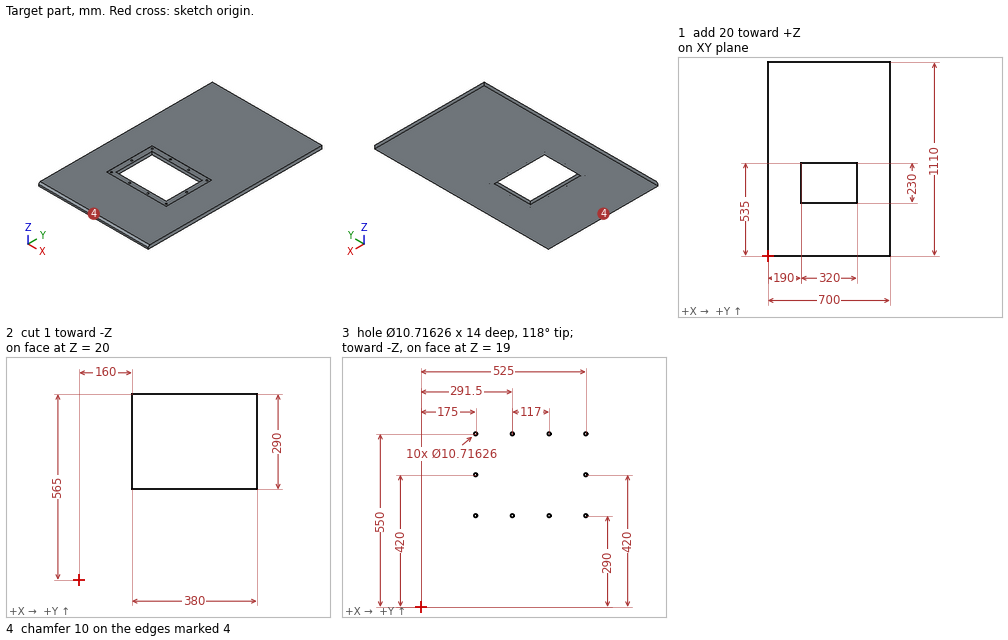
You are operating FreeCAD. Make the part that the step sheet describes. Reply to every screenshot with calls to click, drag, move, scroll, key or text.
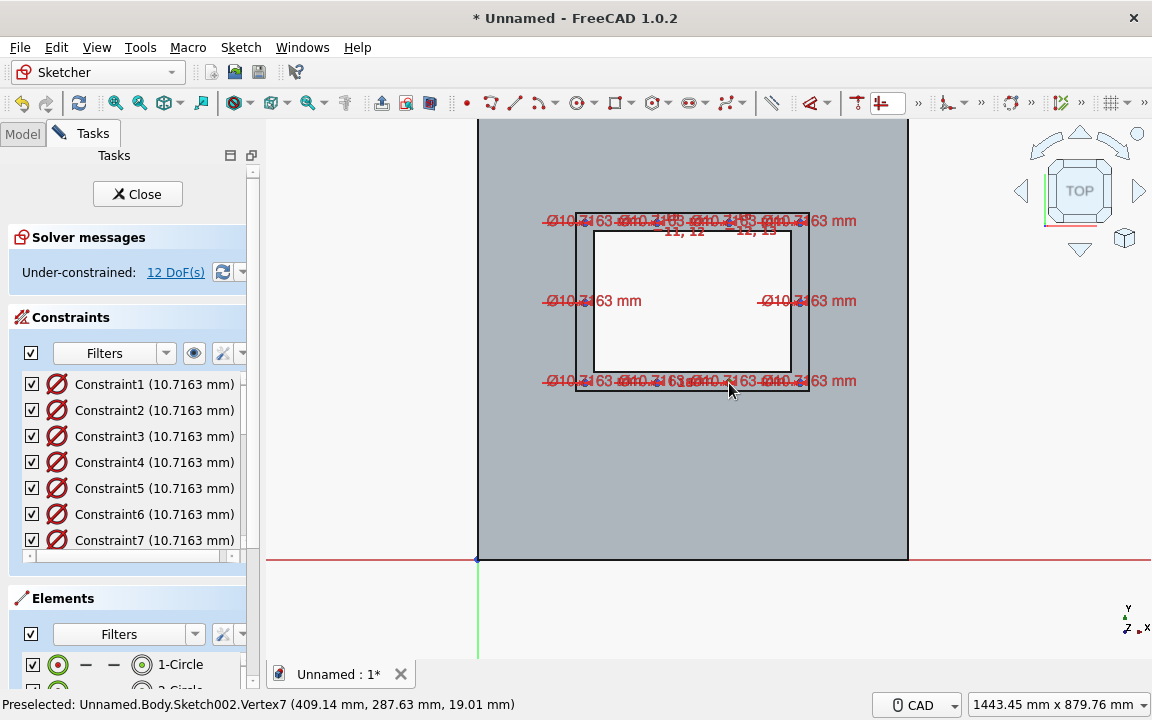
click(657, 383)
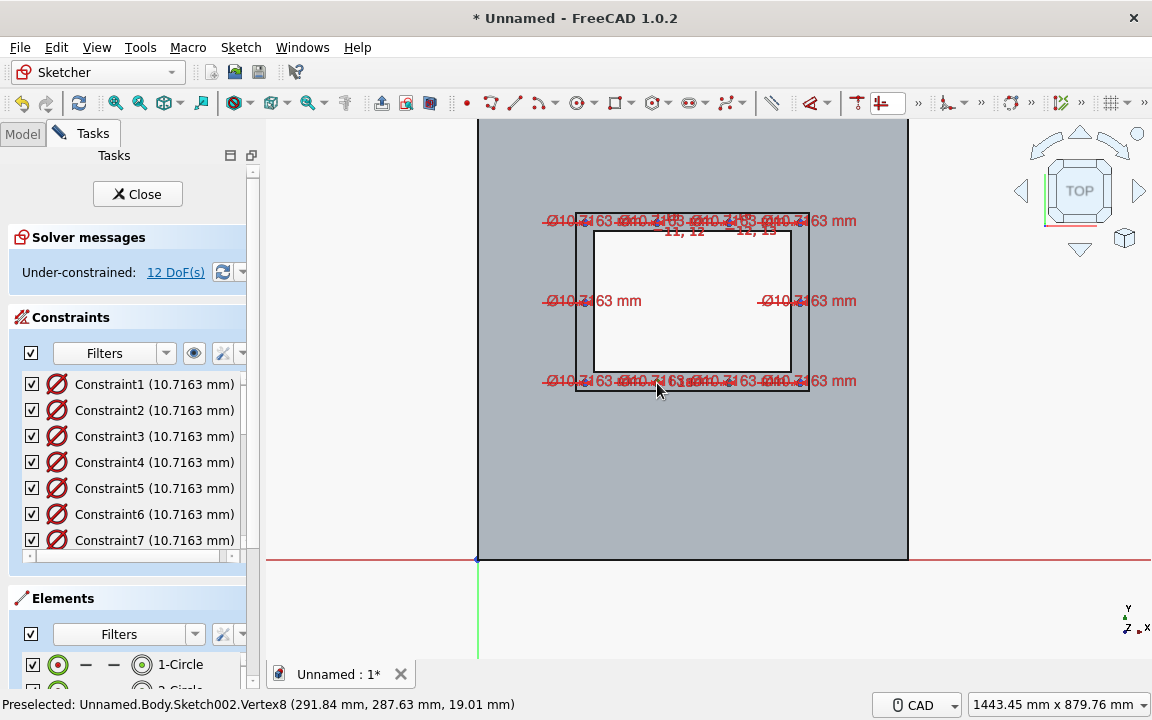
key(h)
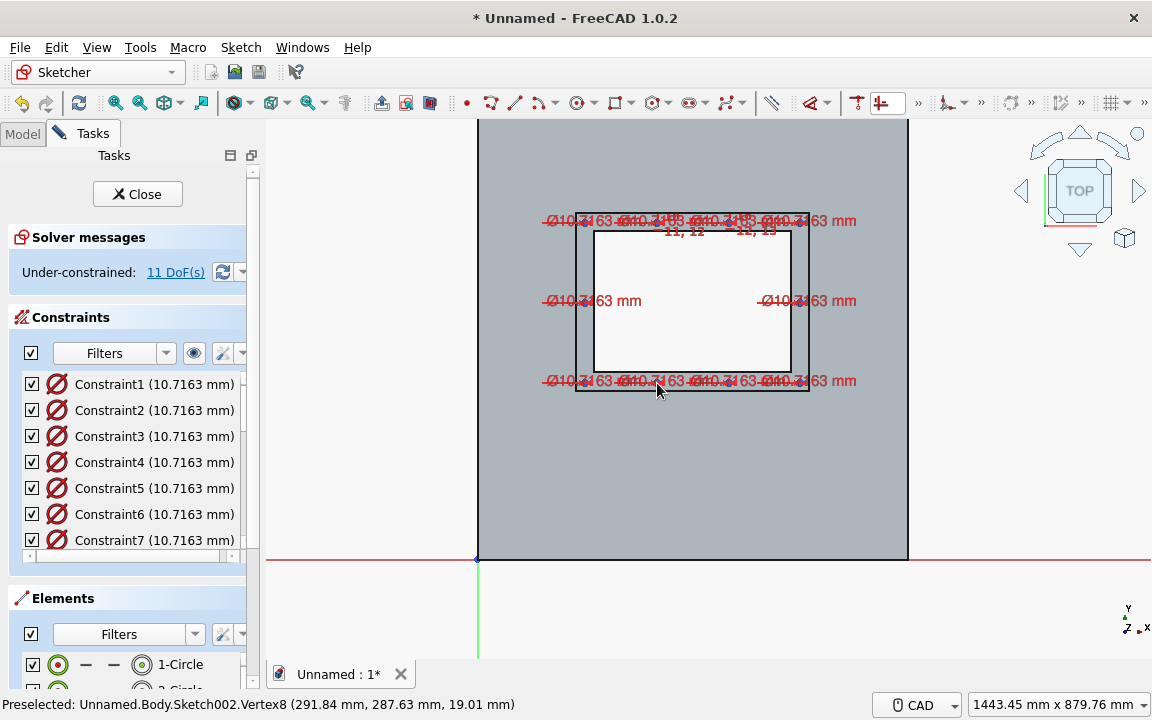
click(585, 223)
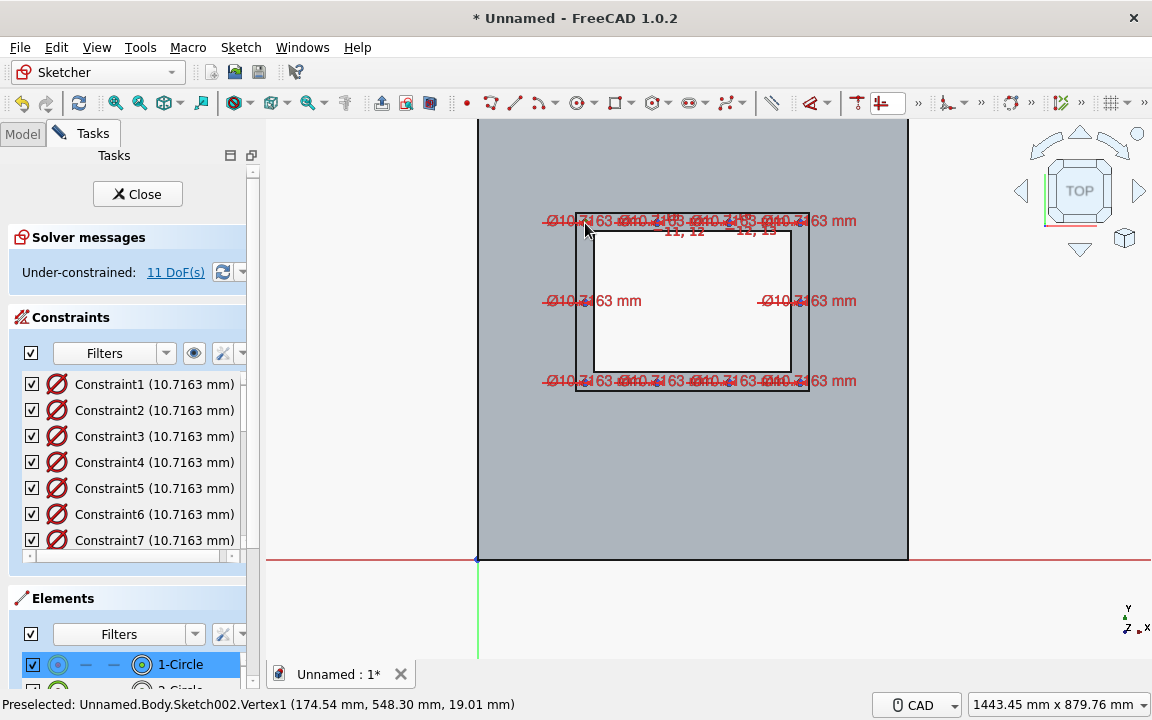
click(585, 383)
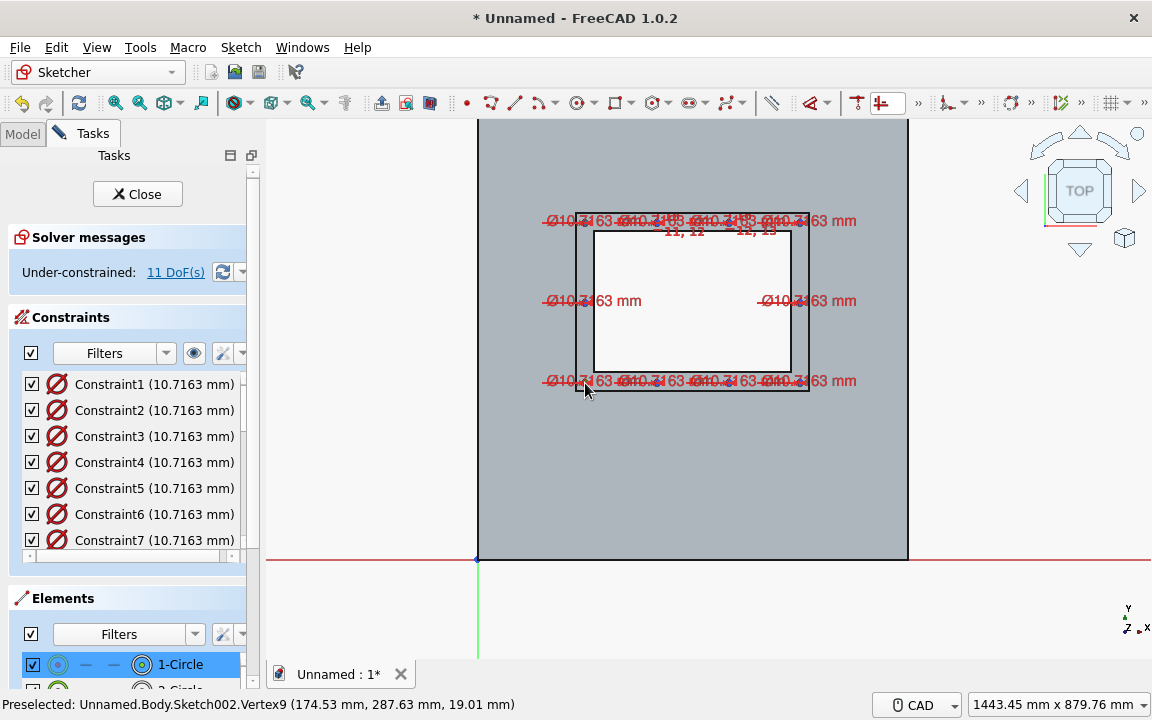
key(v)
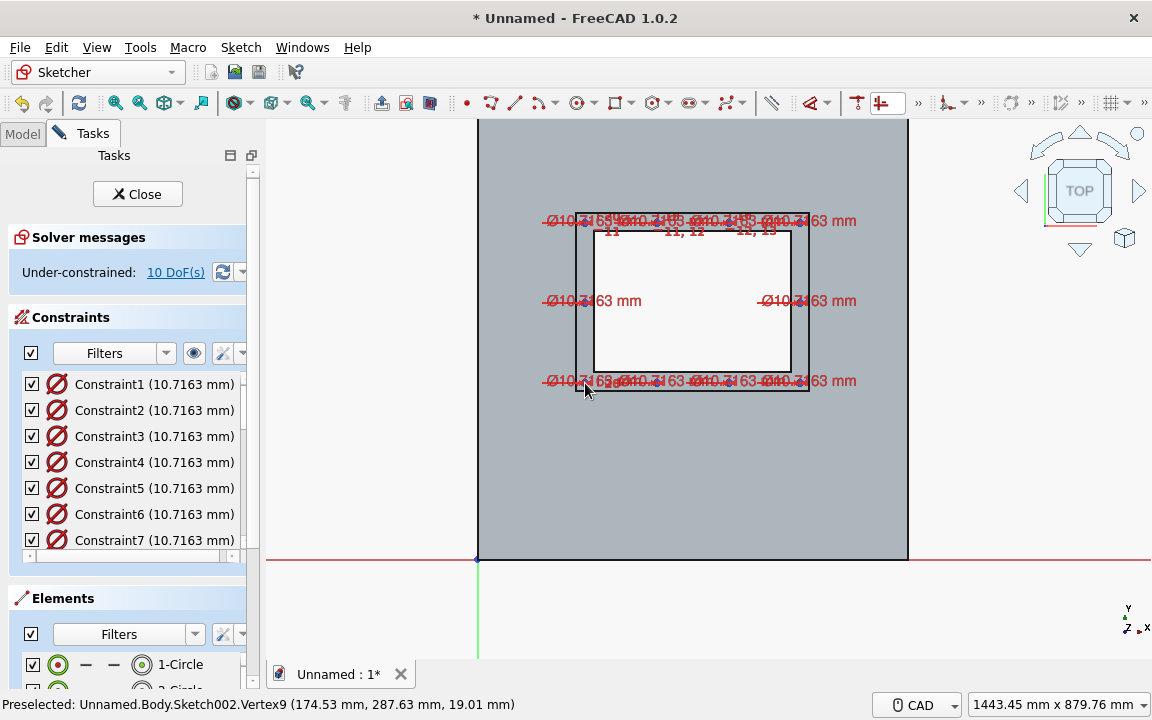
click(657, 383)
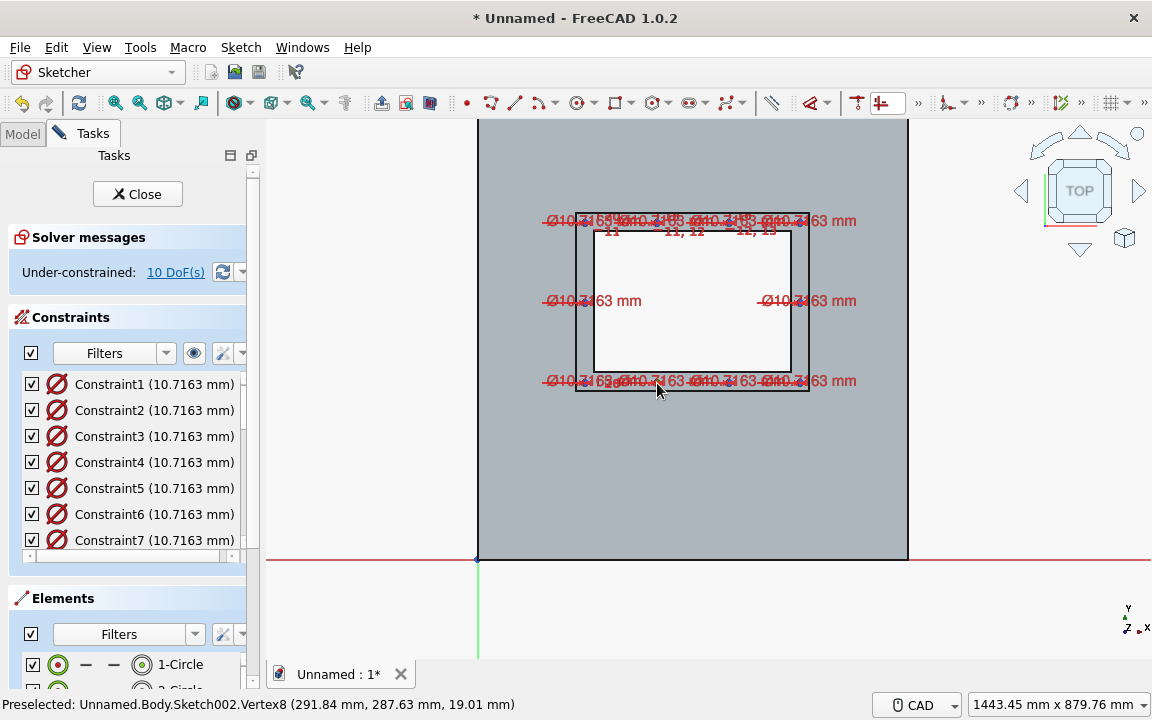
click(585, 383)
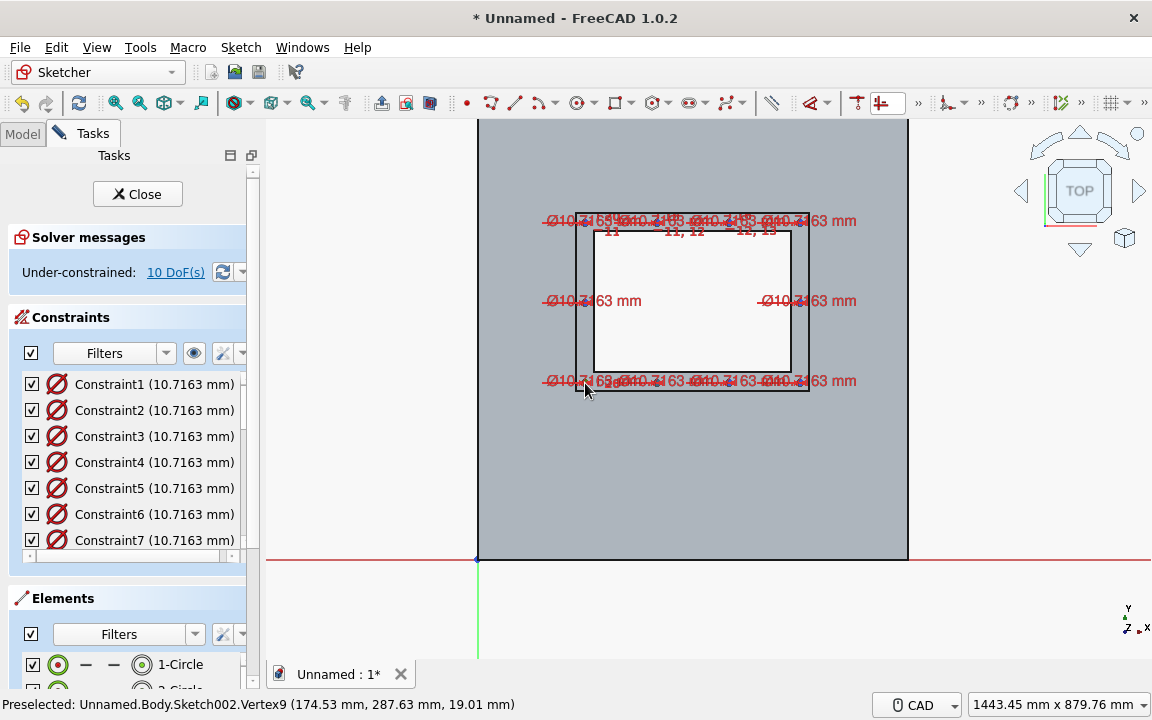
key(h)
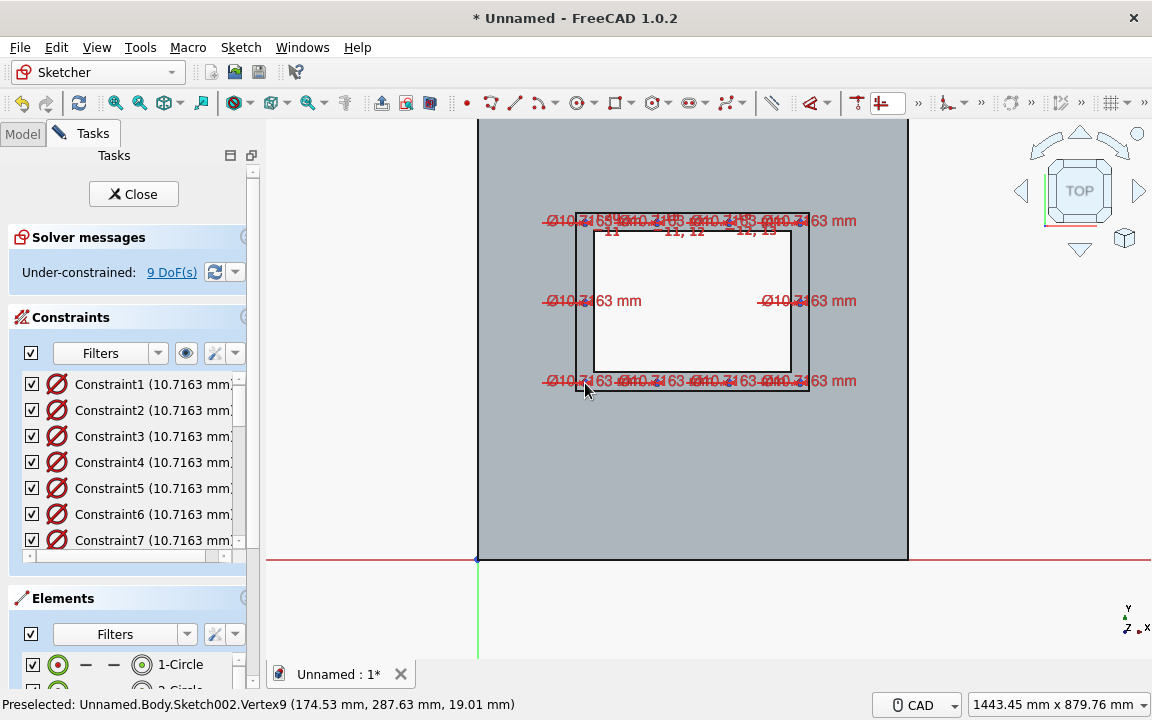
click(585, 223)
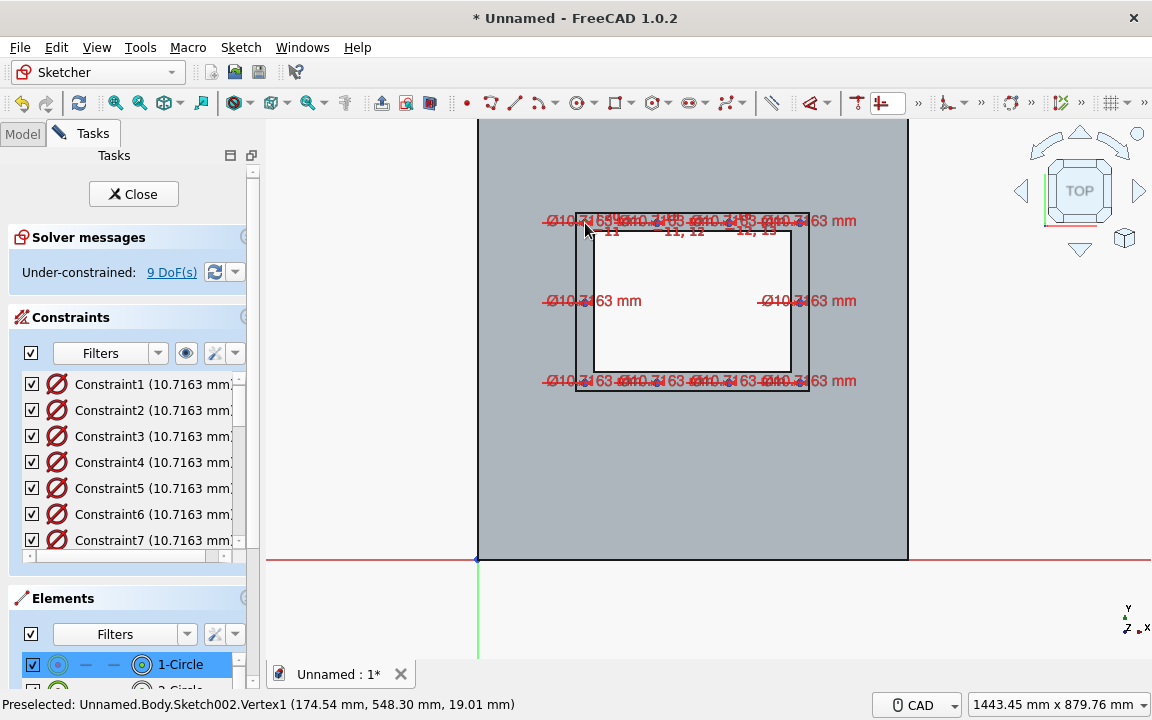
click(585, 303)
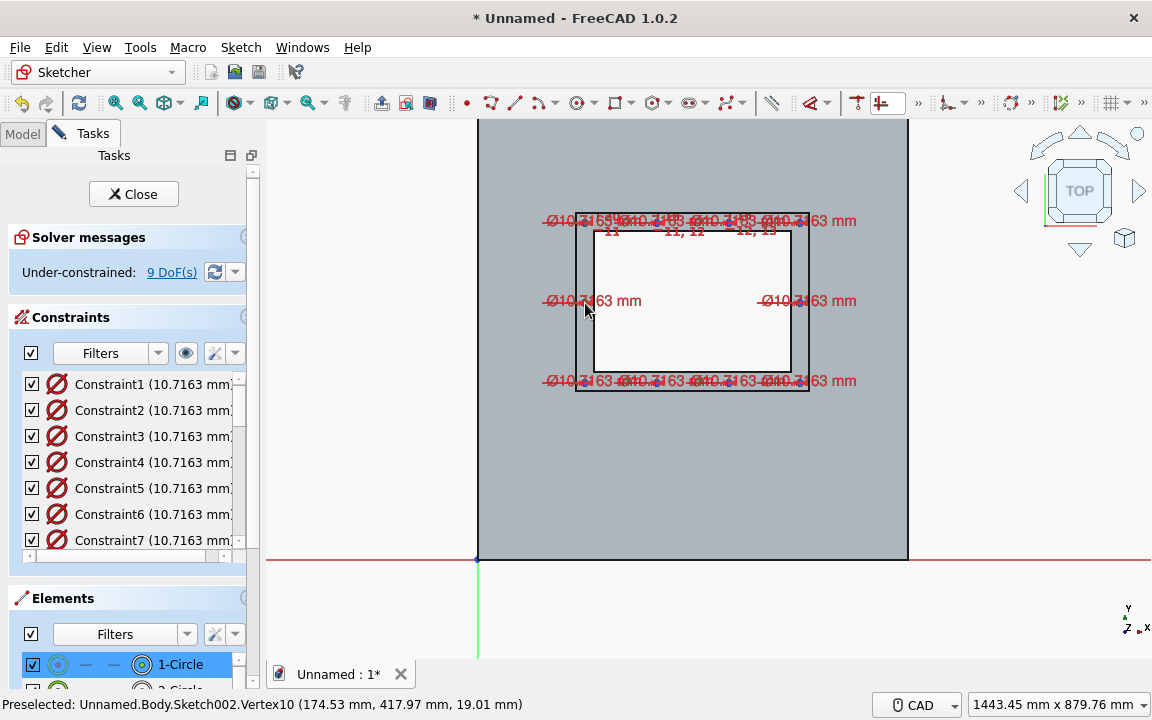
click(900, 104)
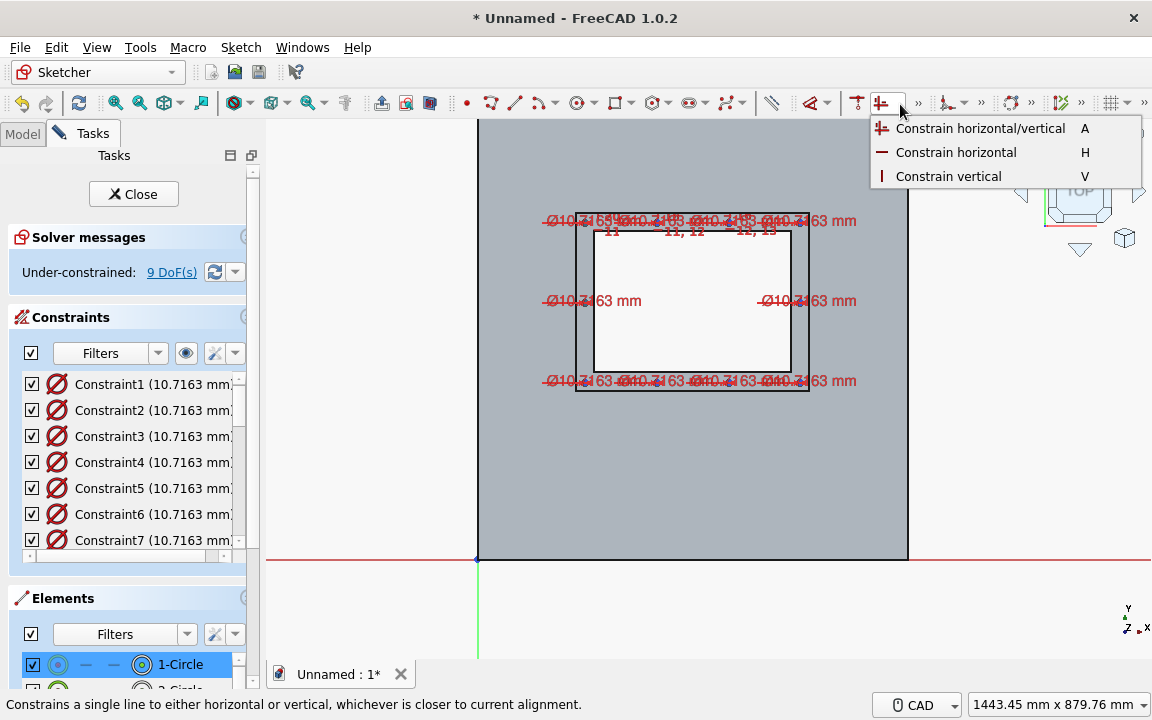
click(1006, 176)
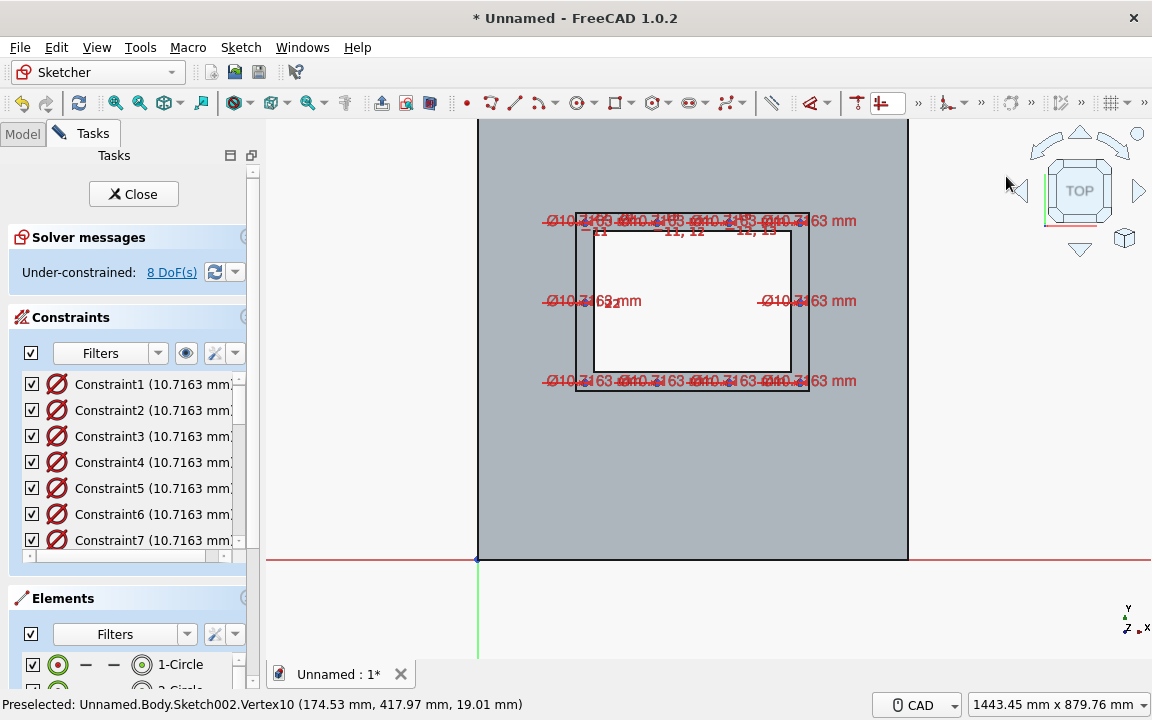
click(810, 104)